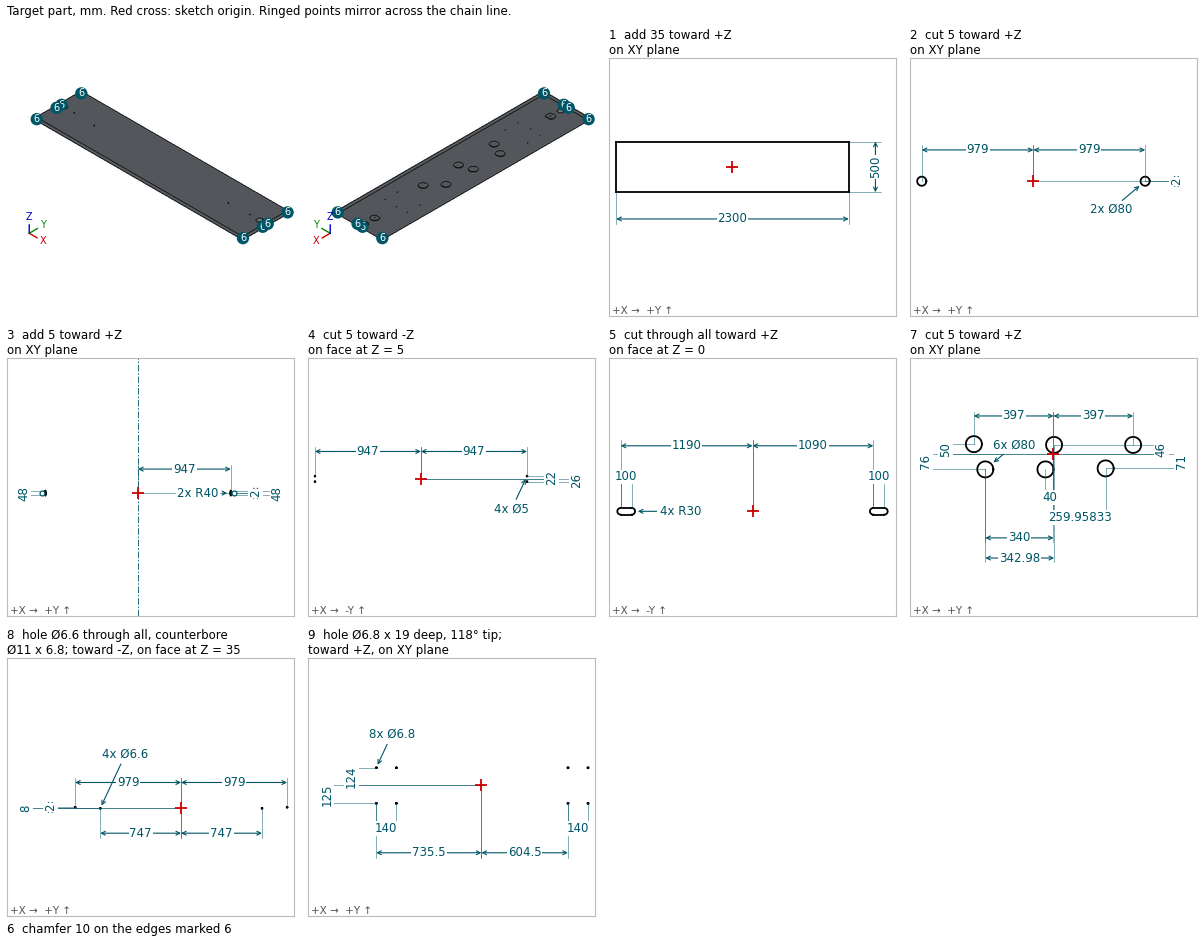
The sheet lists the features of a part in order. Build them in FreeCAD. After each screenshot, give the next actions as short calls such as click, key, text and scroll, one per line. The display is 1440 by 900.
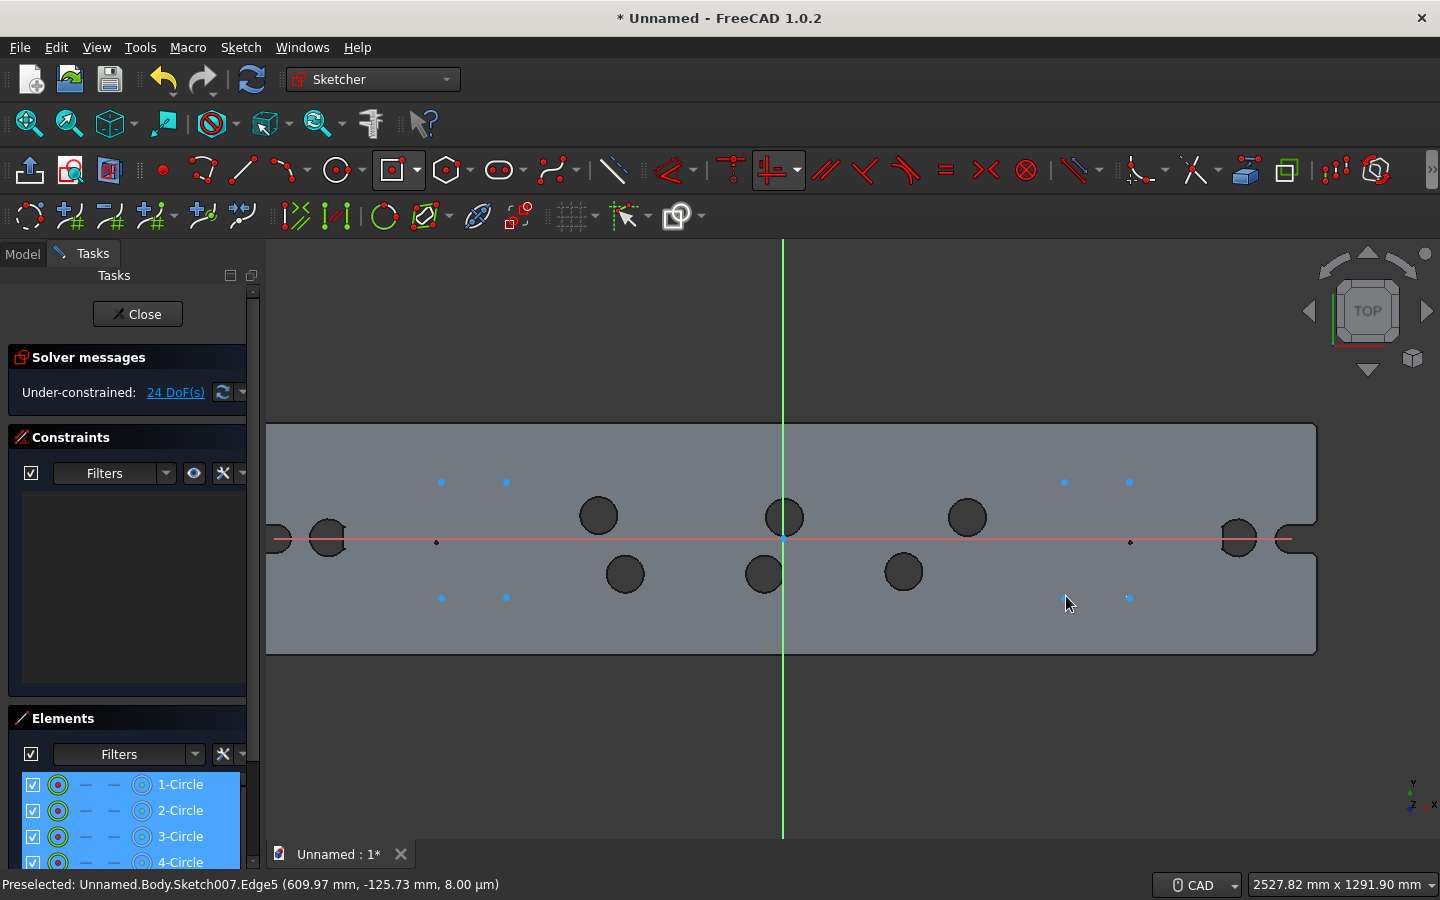
scroll(1131, 596, up, 9)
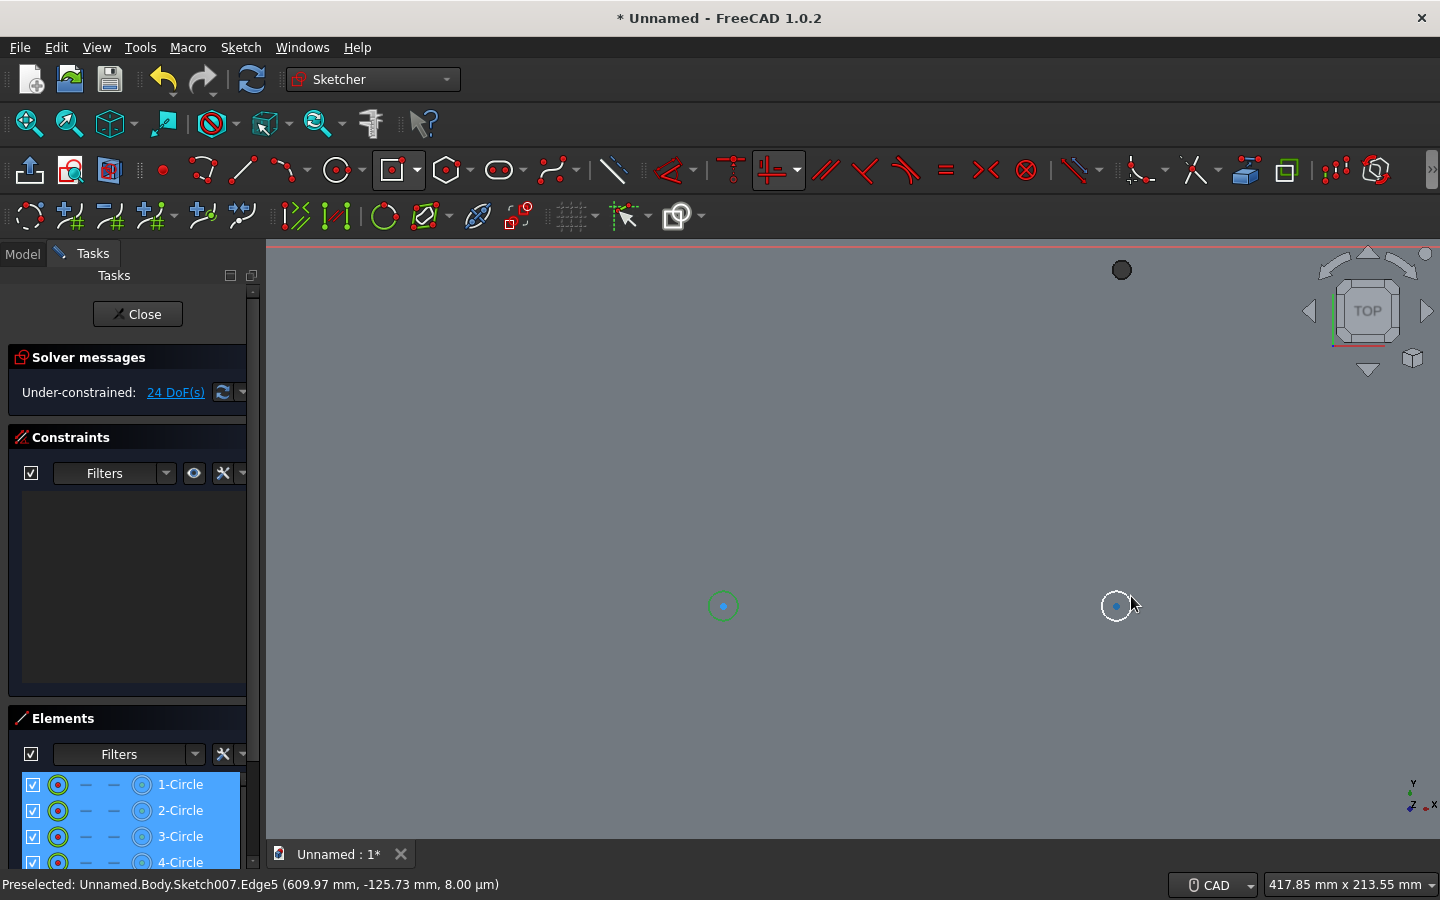
click(1127, 596)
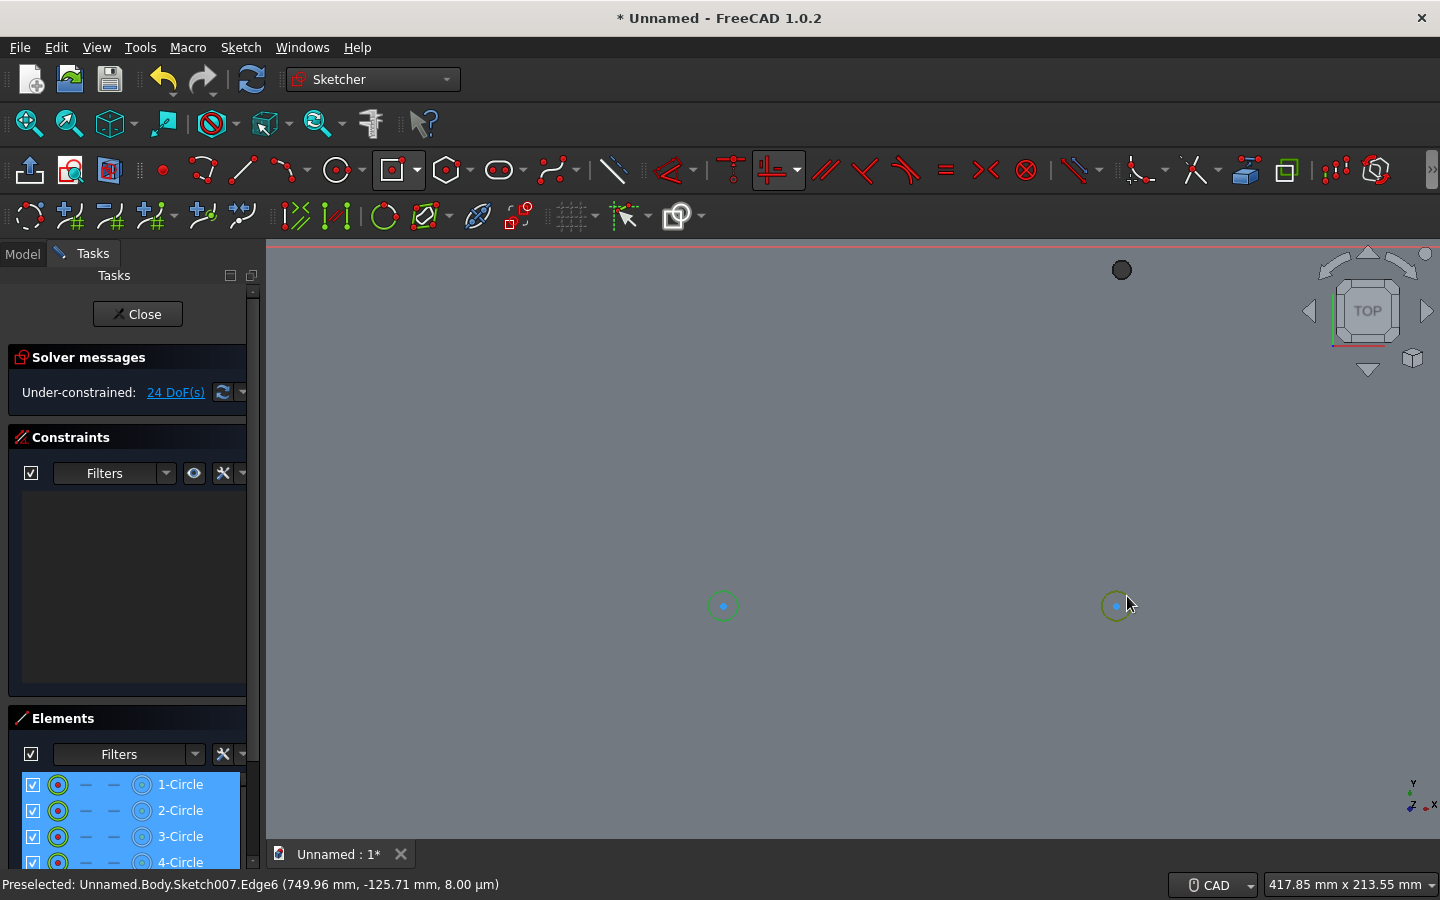
scroll(1131, 596, down, 9)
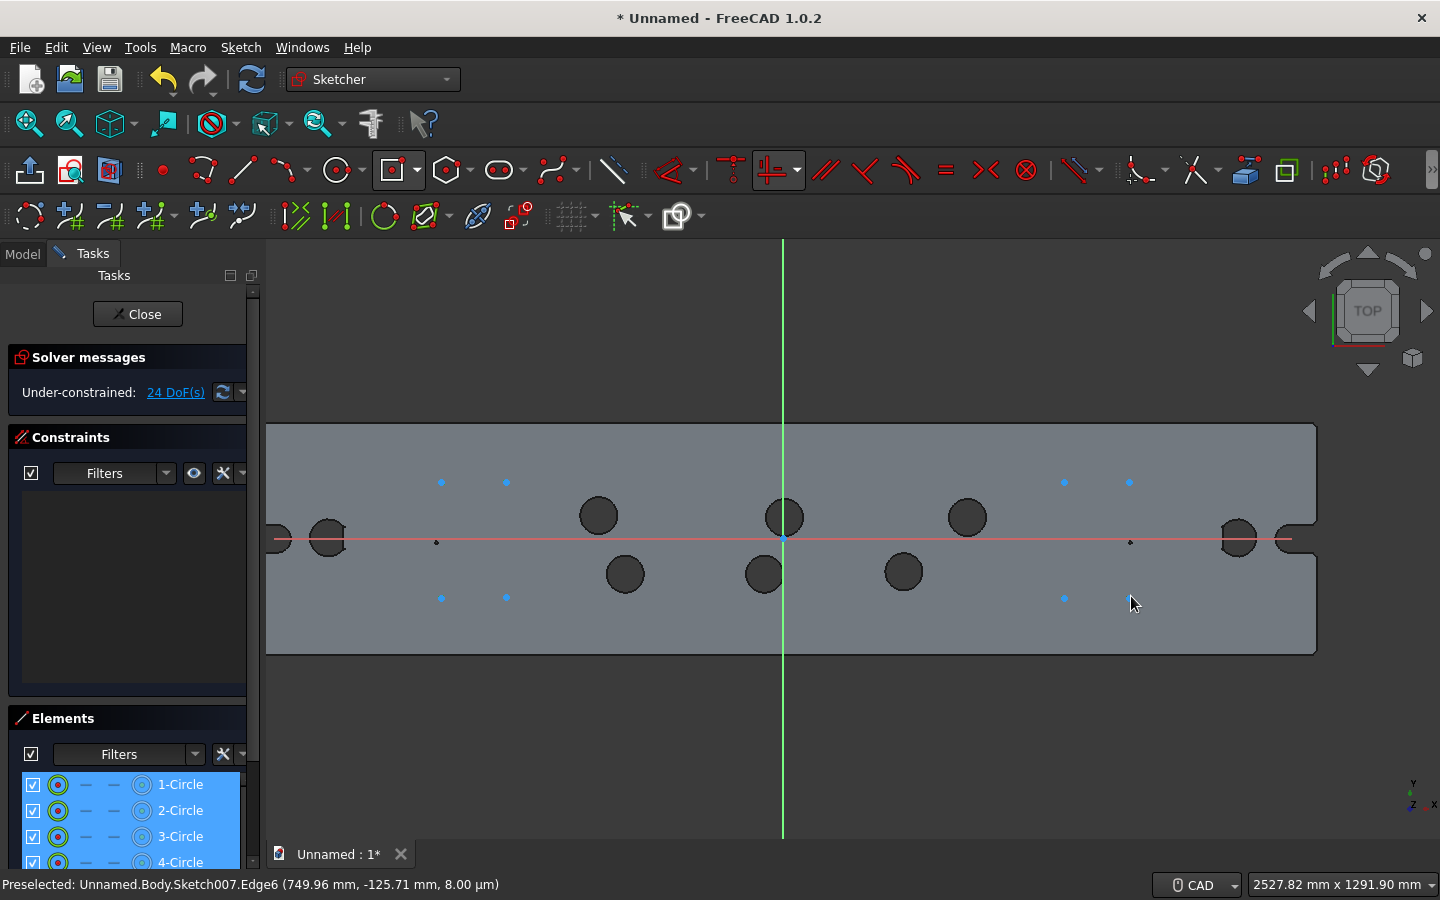
scroll(1066, 481, up, 10)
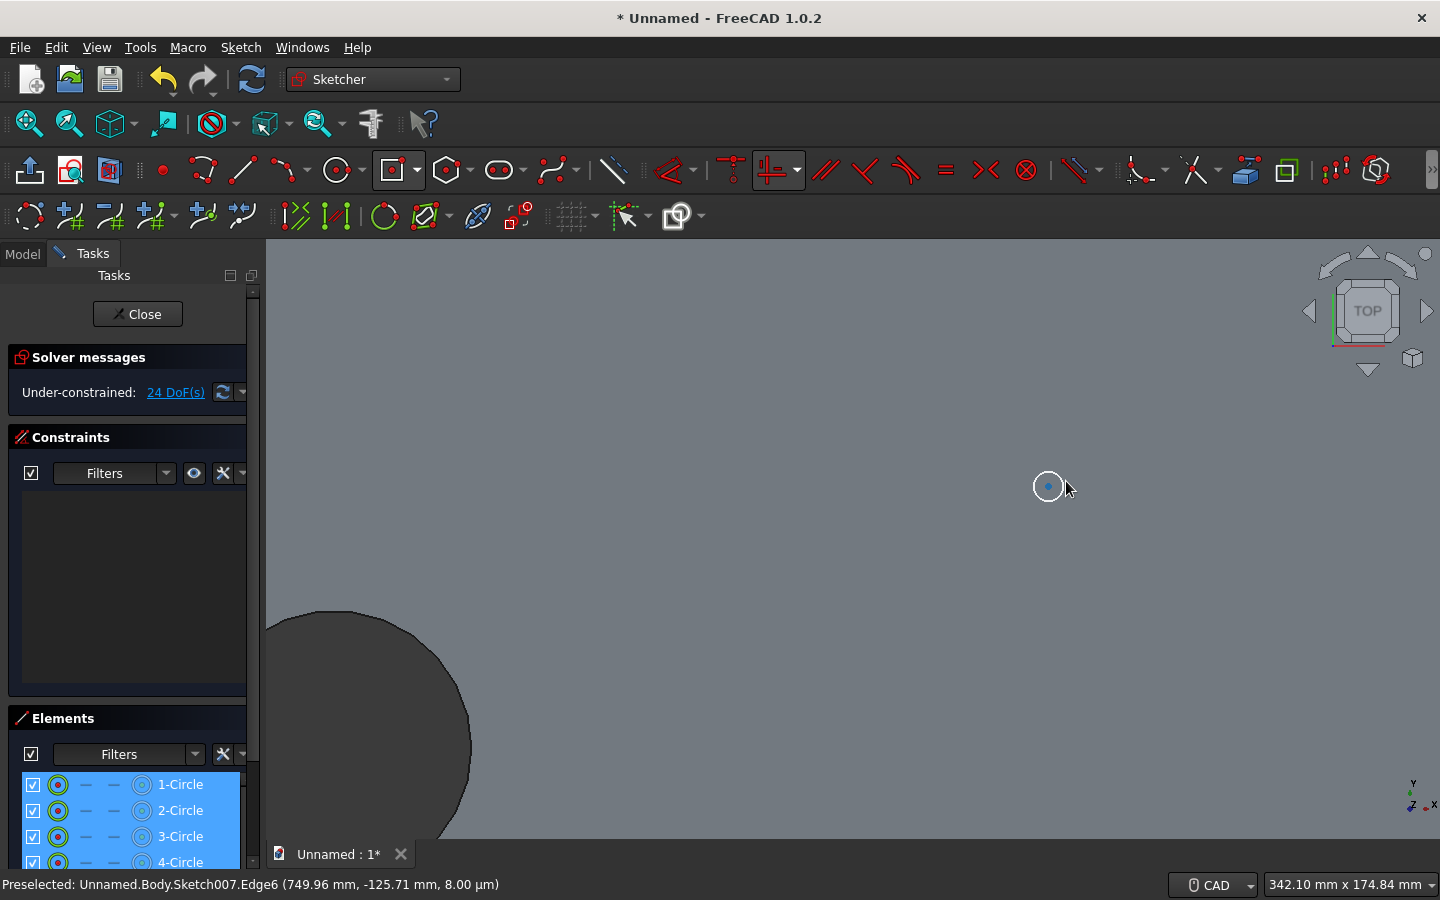
click(1059, 476)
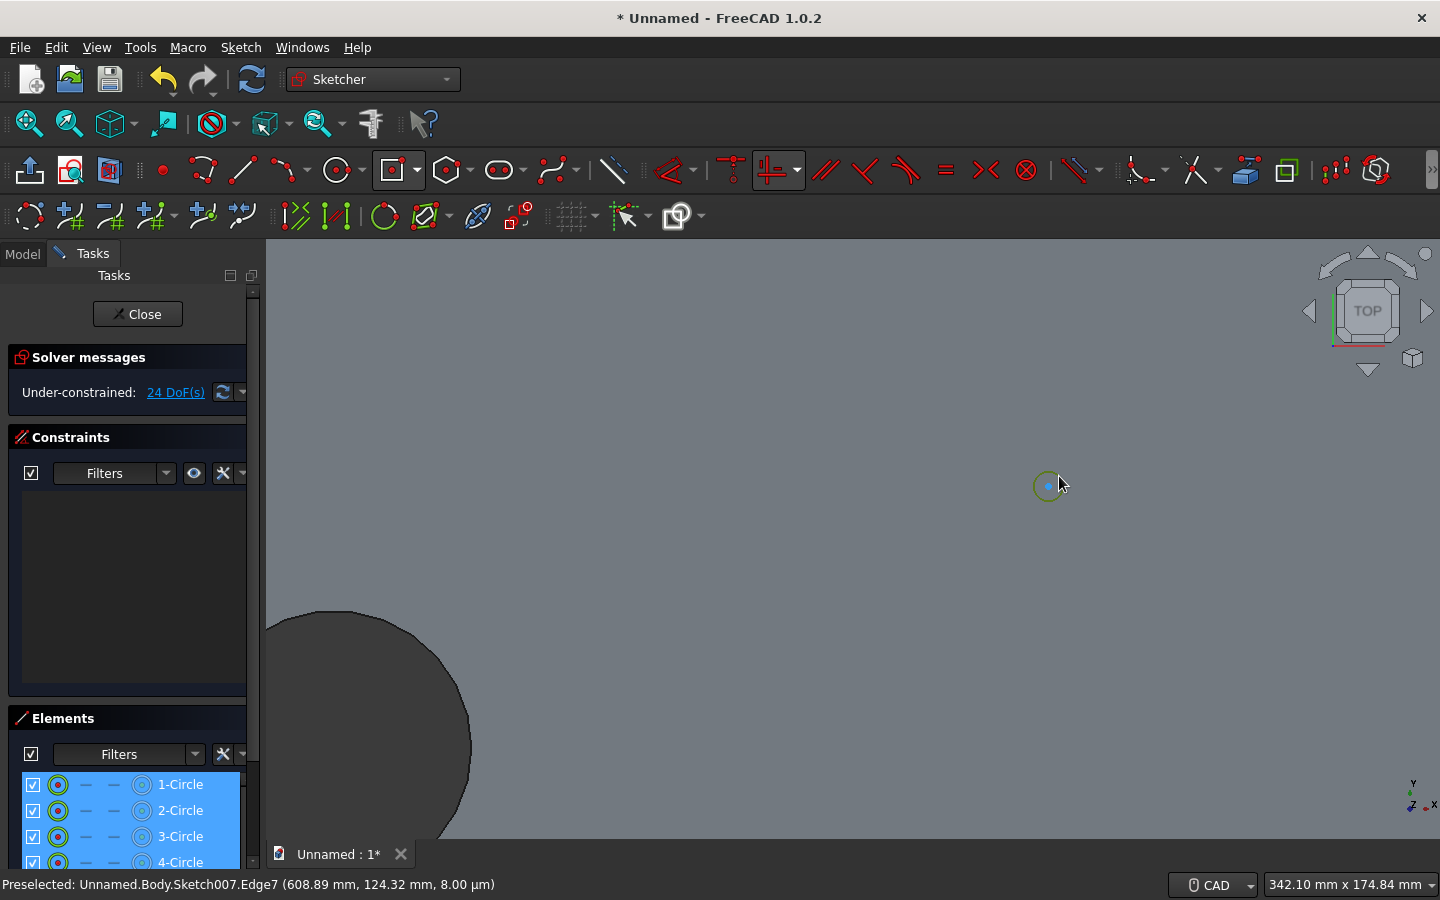
scroll(1066, 481, down, 10)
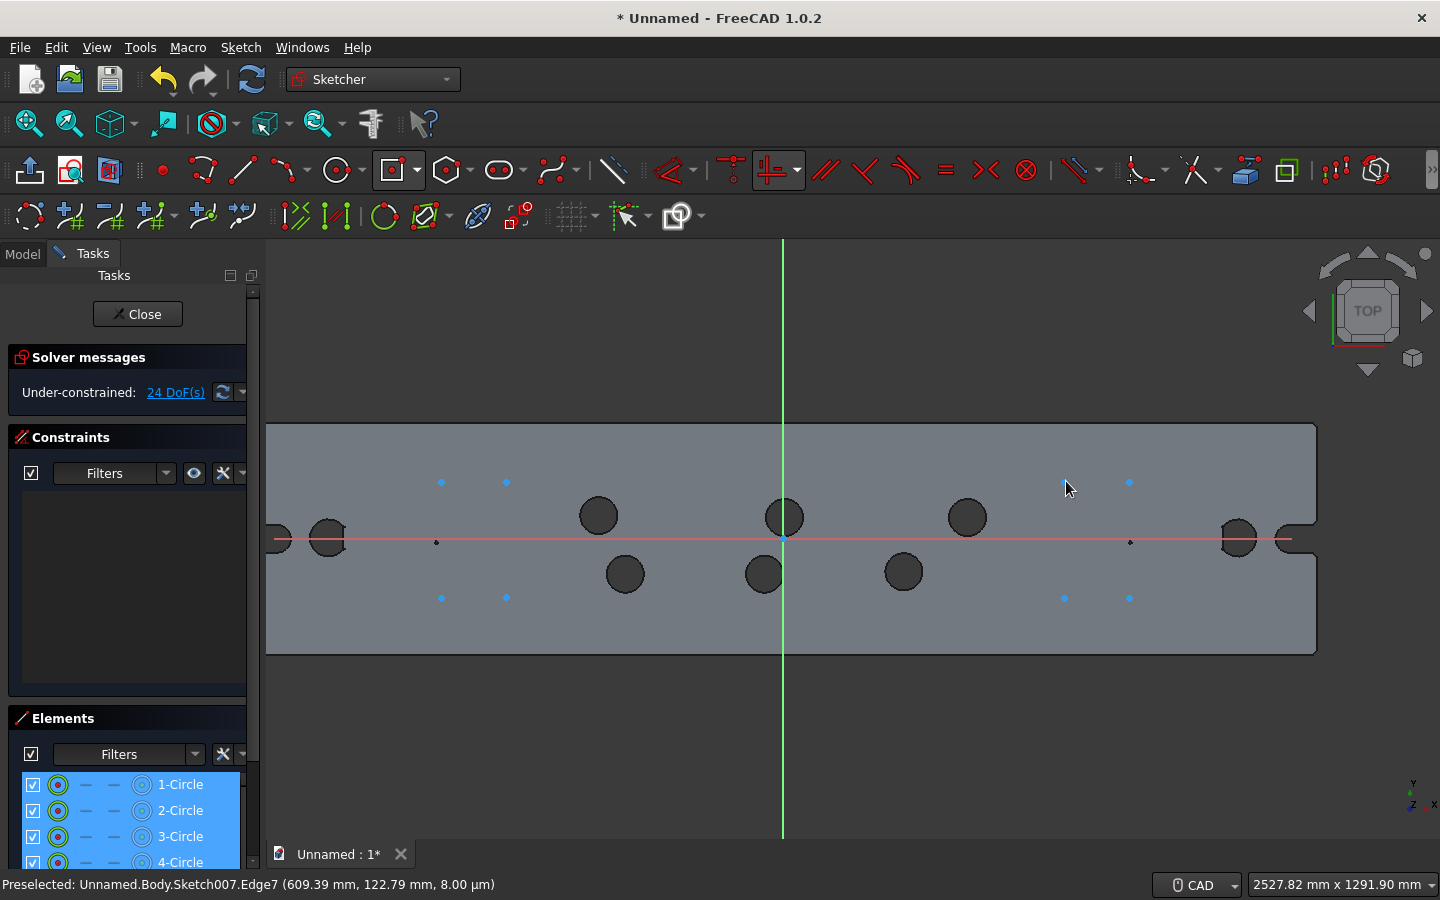
scroll(1131, 481, up, 10)